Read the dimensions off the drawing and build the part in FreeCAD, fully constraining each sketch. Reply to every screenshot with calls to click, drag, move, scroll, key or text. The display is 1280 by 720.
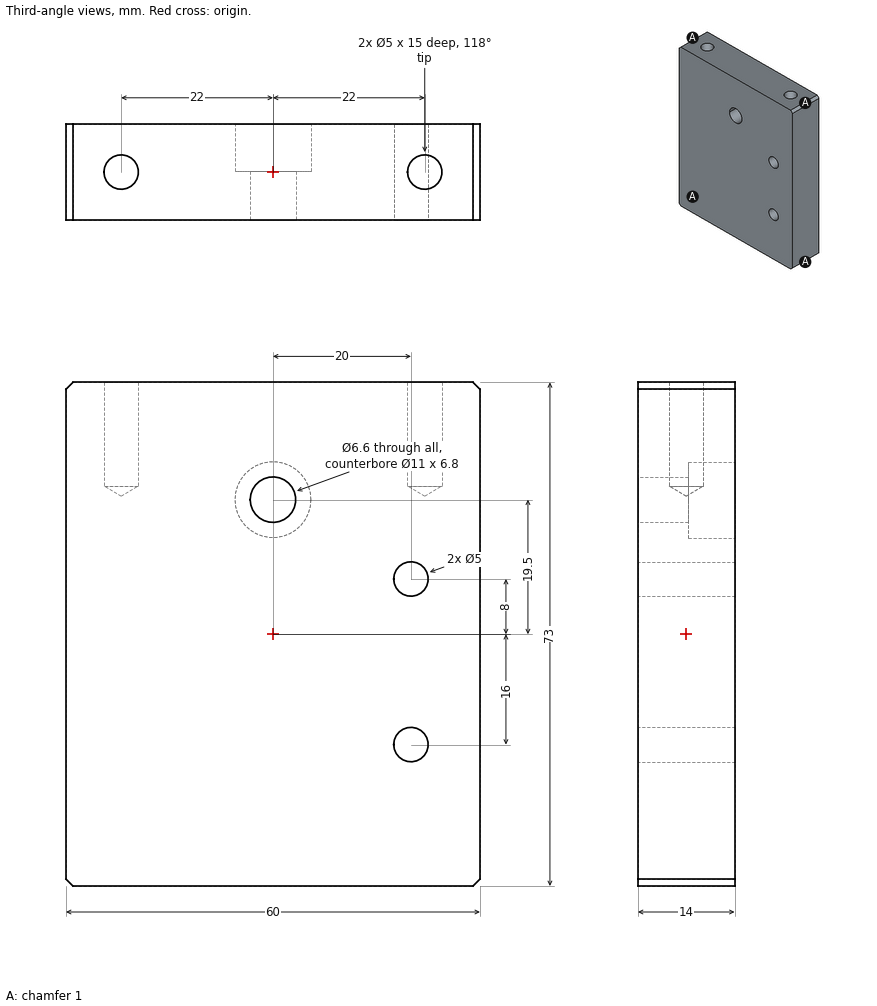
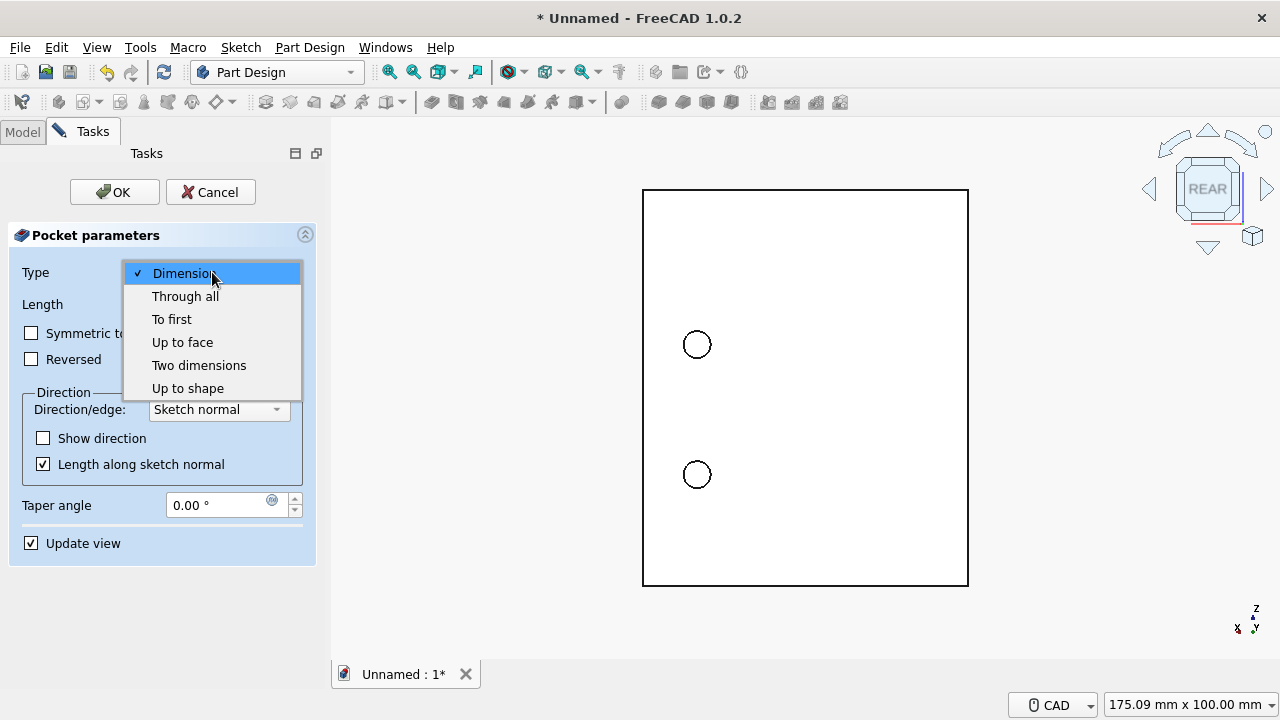
click(212, 296)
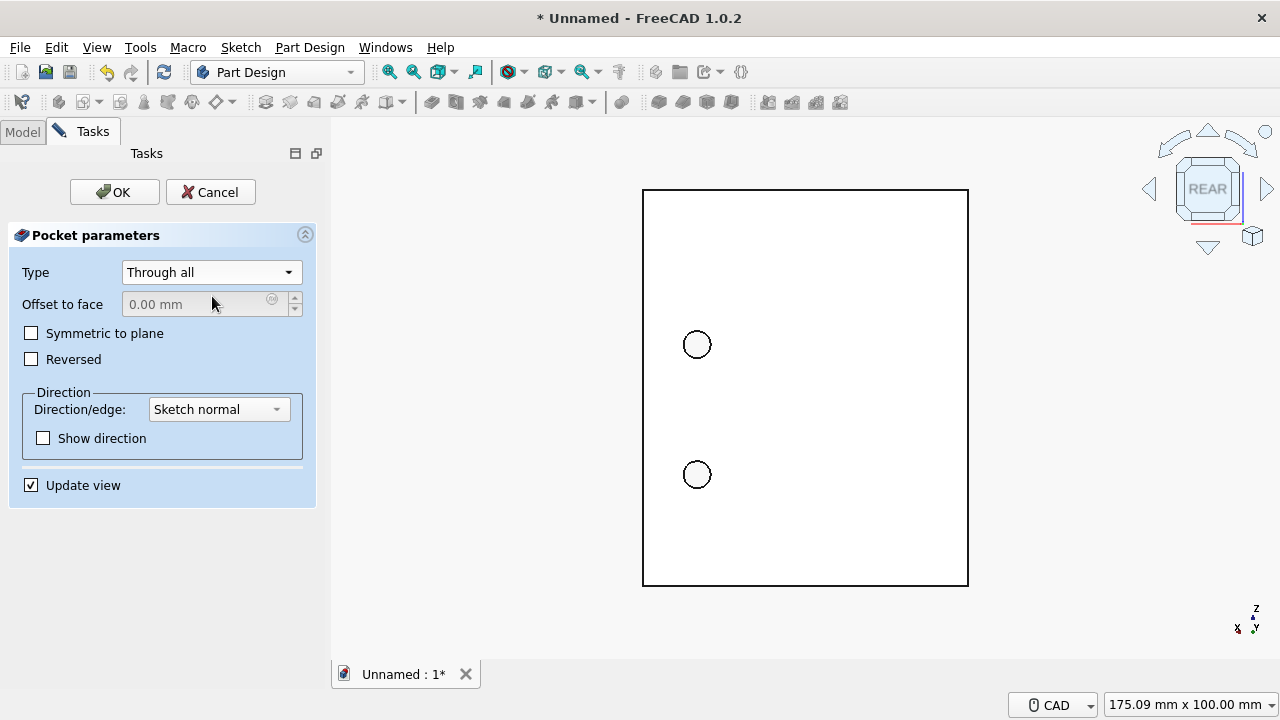
click(115, 192)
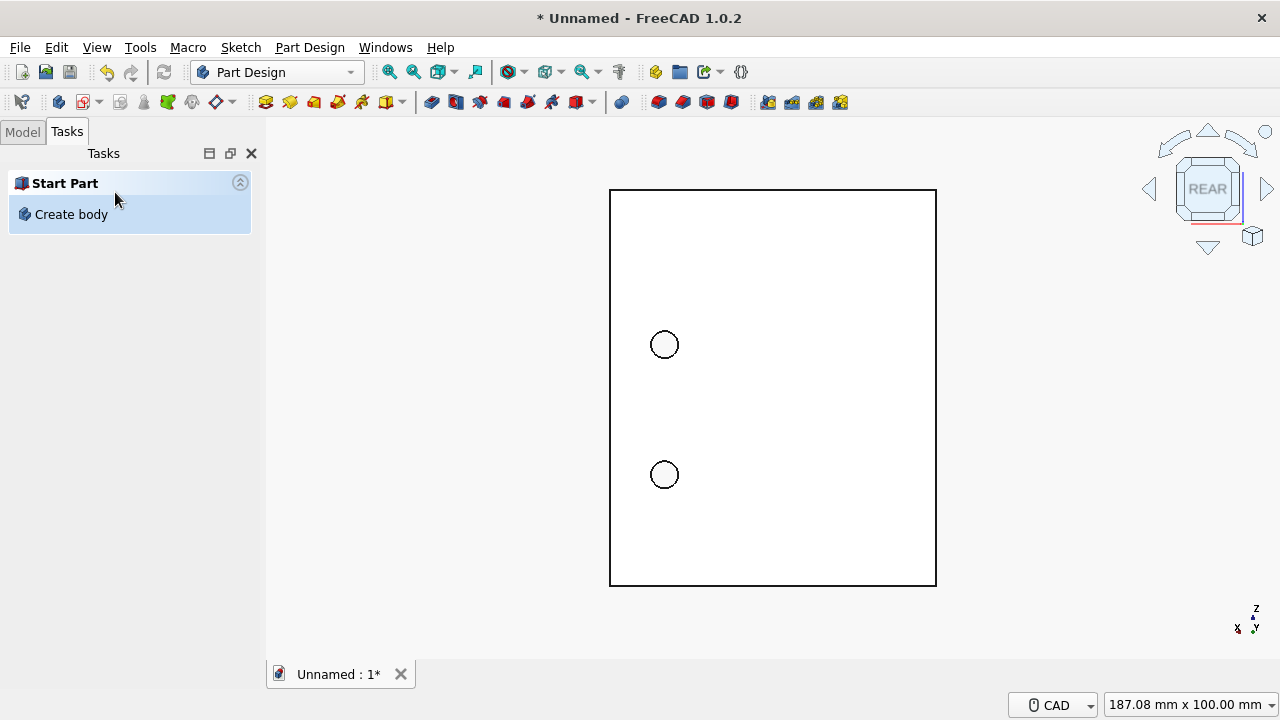
key(0)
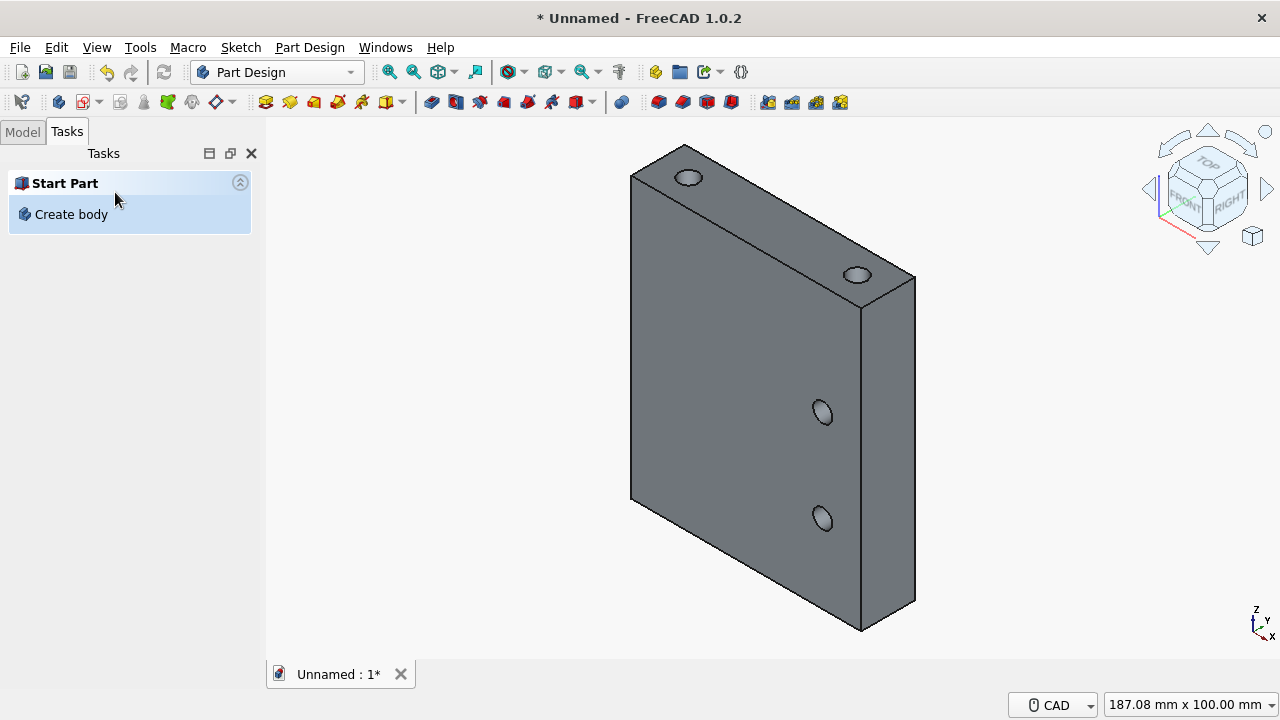
click(888, 292)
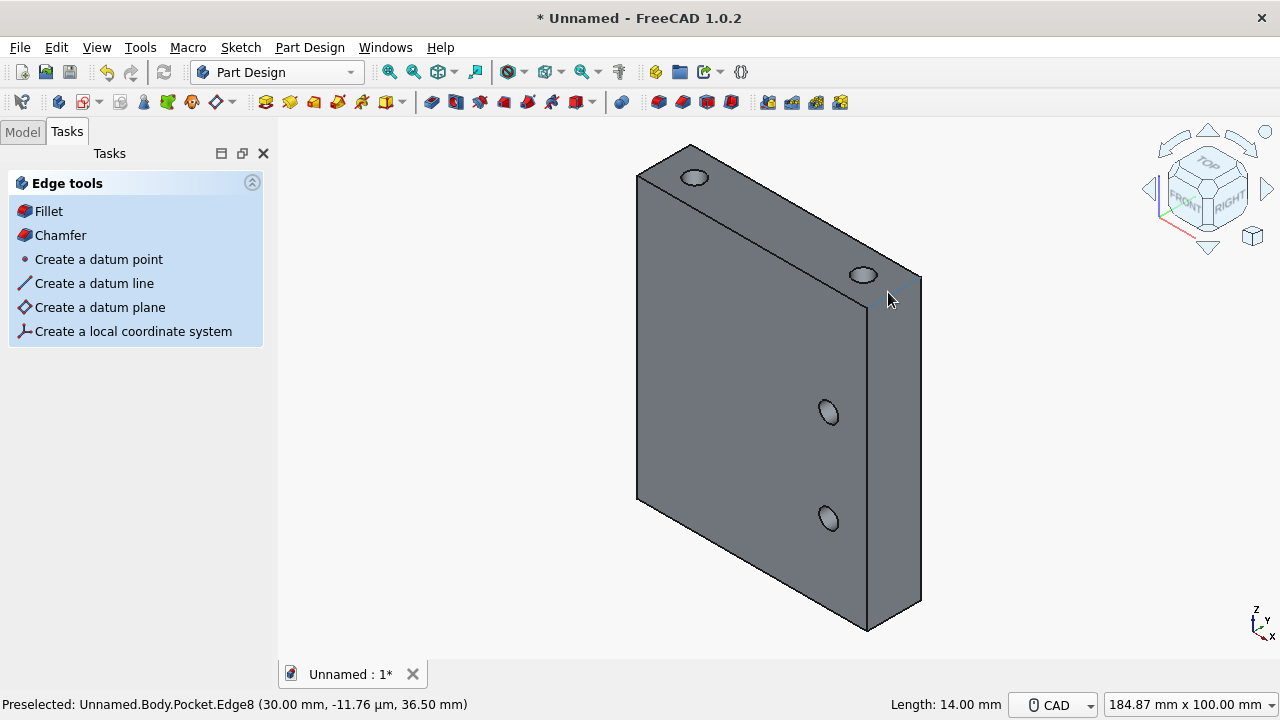
key(2)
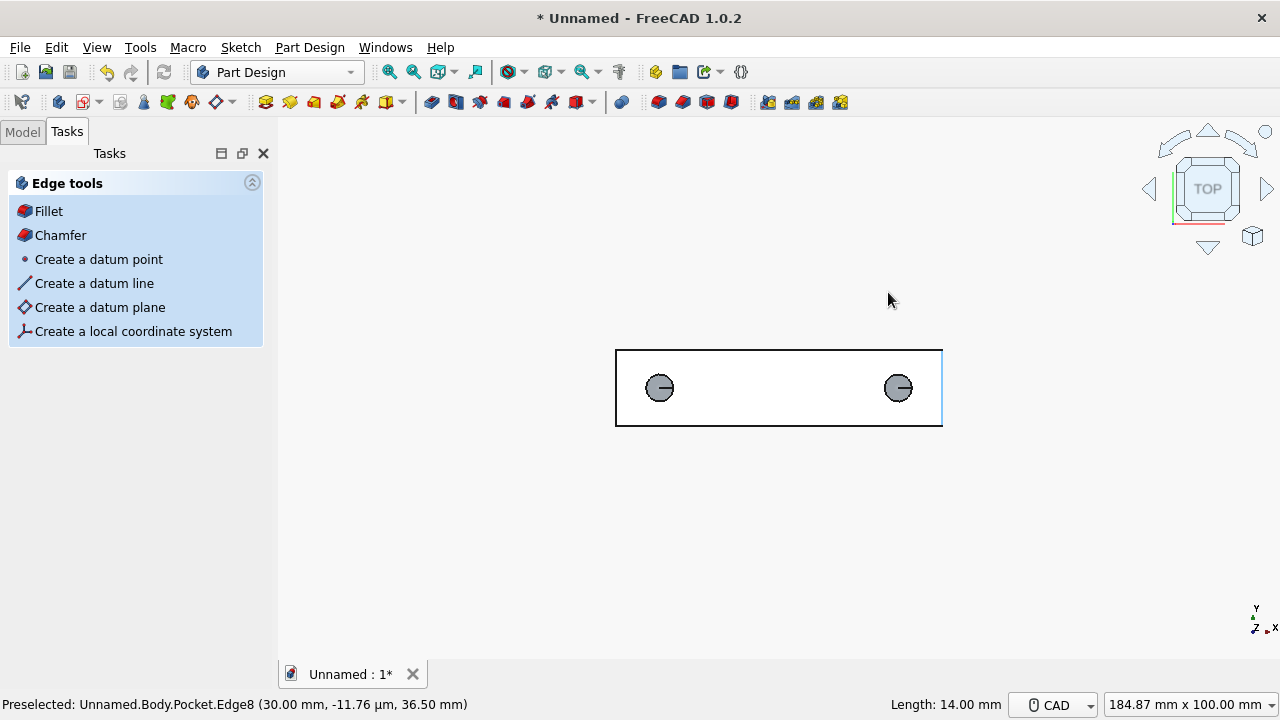
click(390, 72)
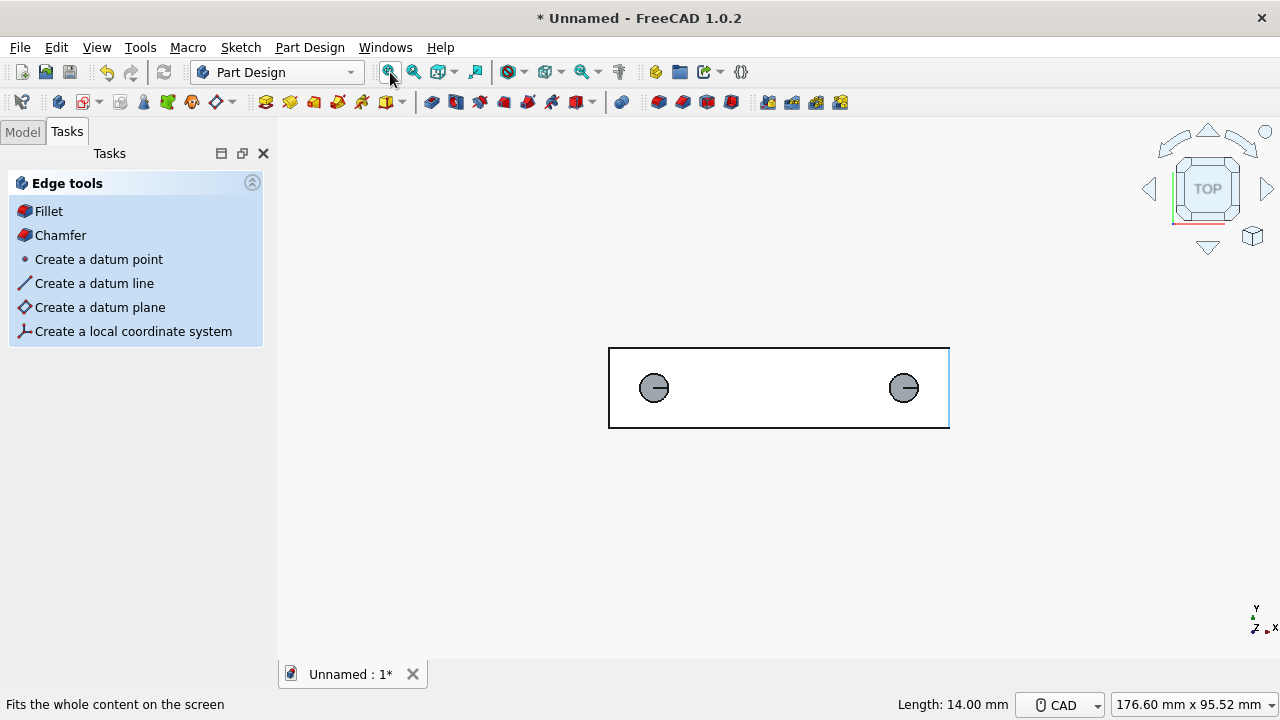
click(609, 387, ctrl)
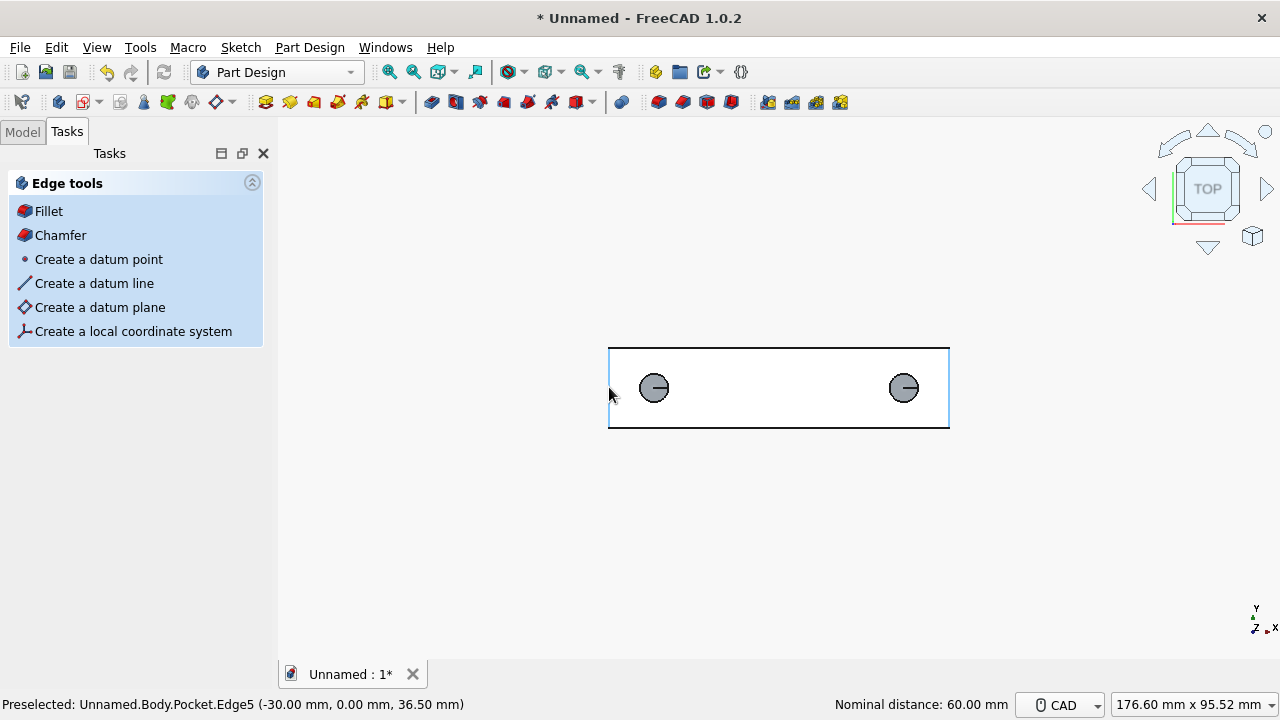
key(1)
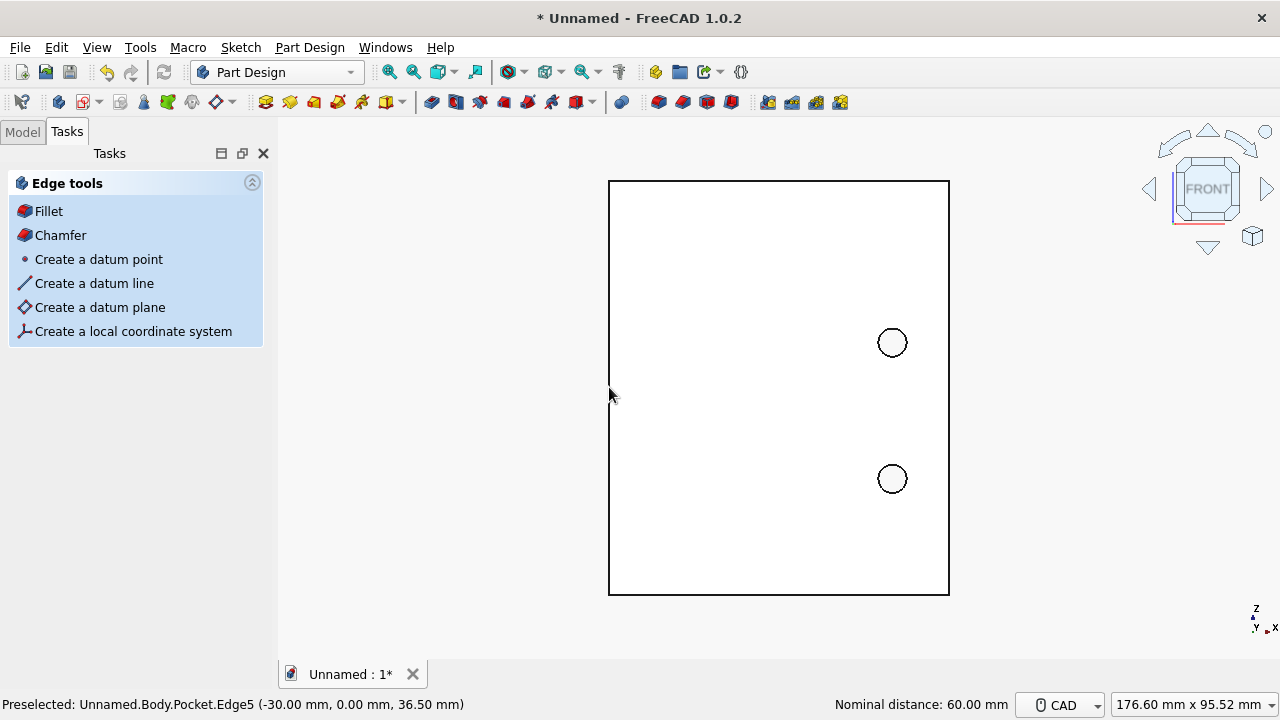
key(3)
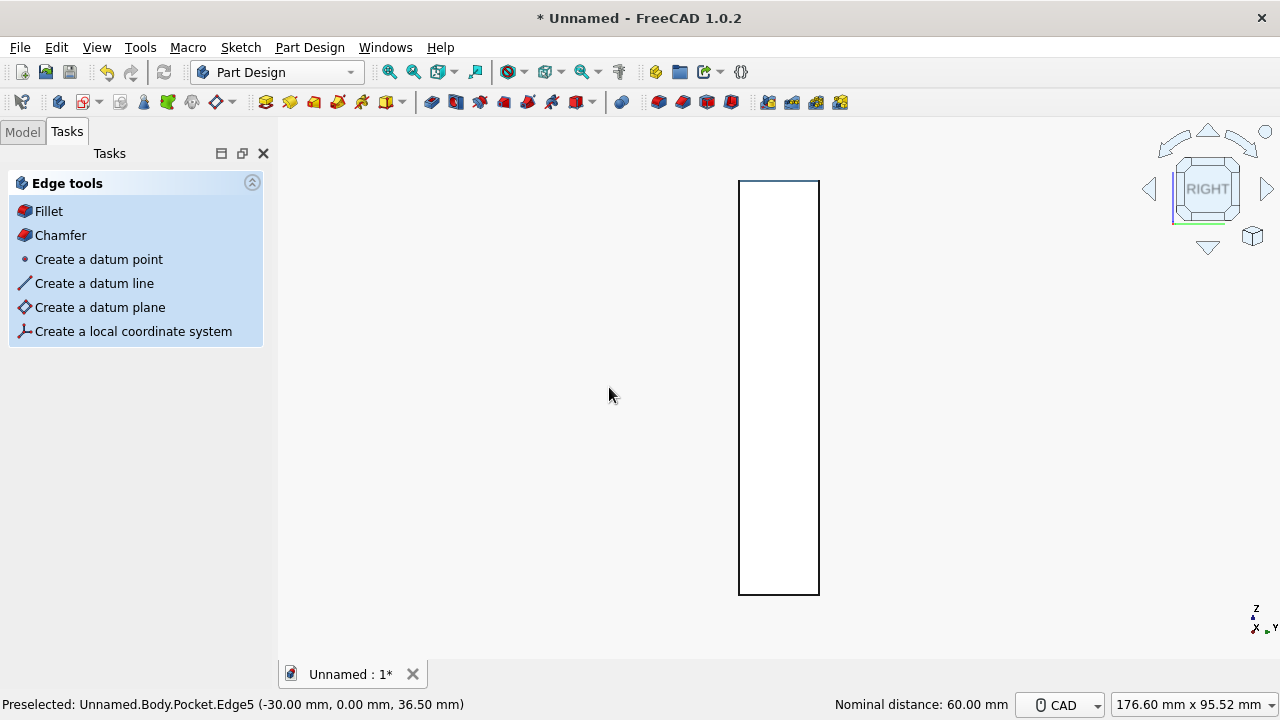
click(779, 594, ctrl)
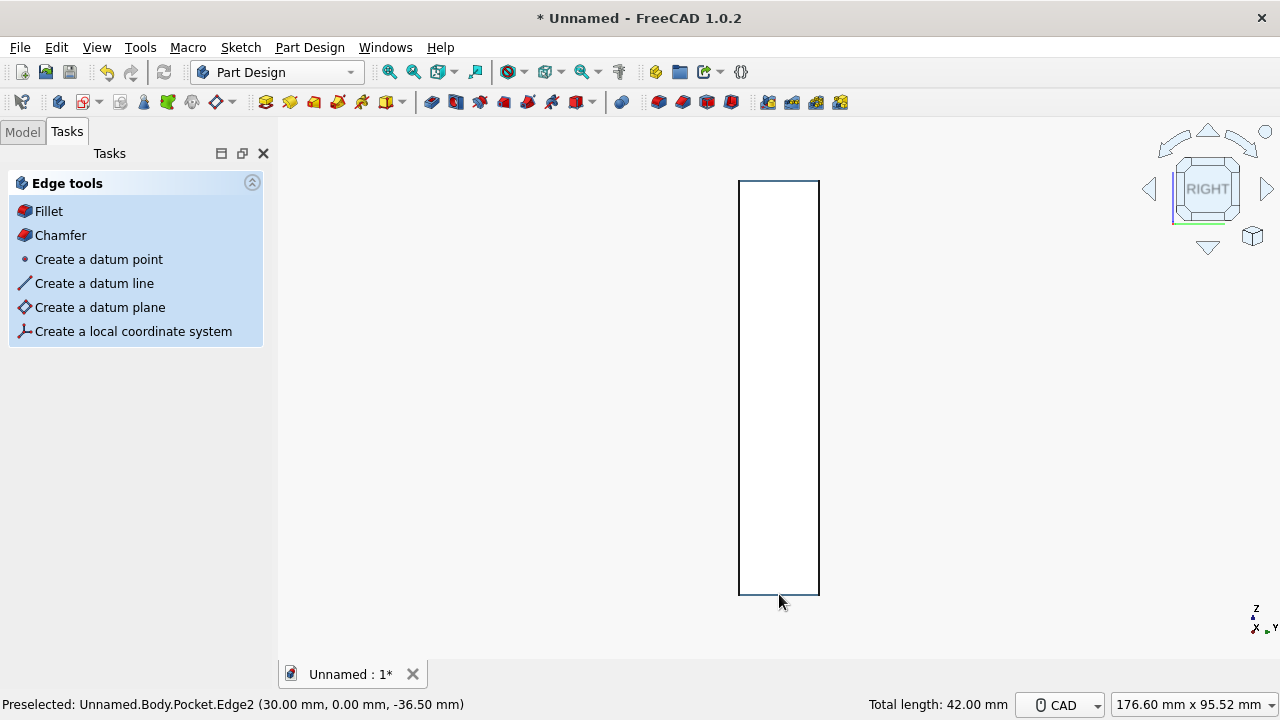
key(5)